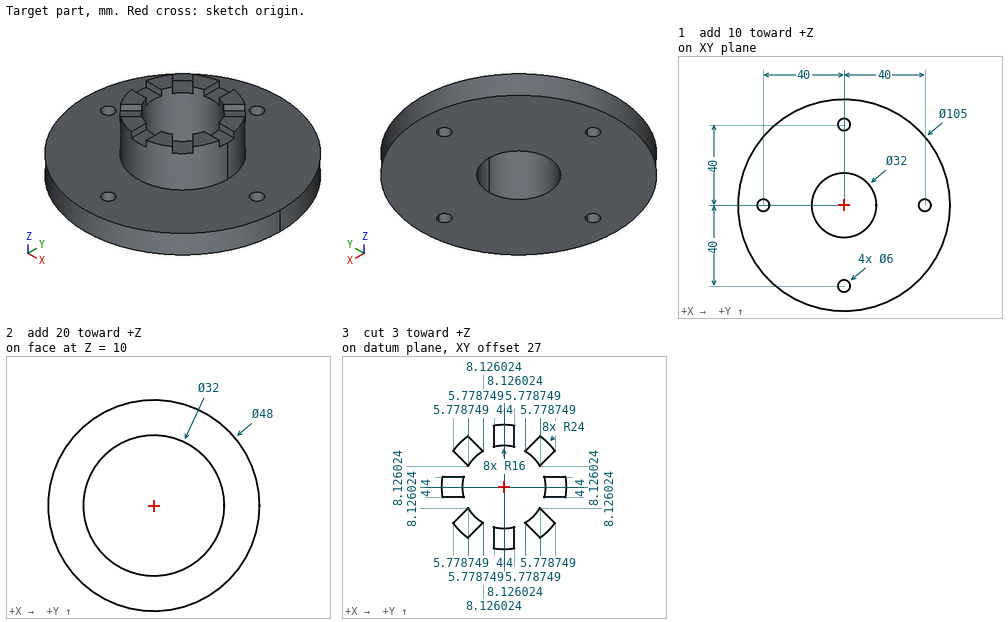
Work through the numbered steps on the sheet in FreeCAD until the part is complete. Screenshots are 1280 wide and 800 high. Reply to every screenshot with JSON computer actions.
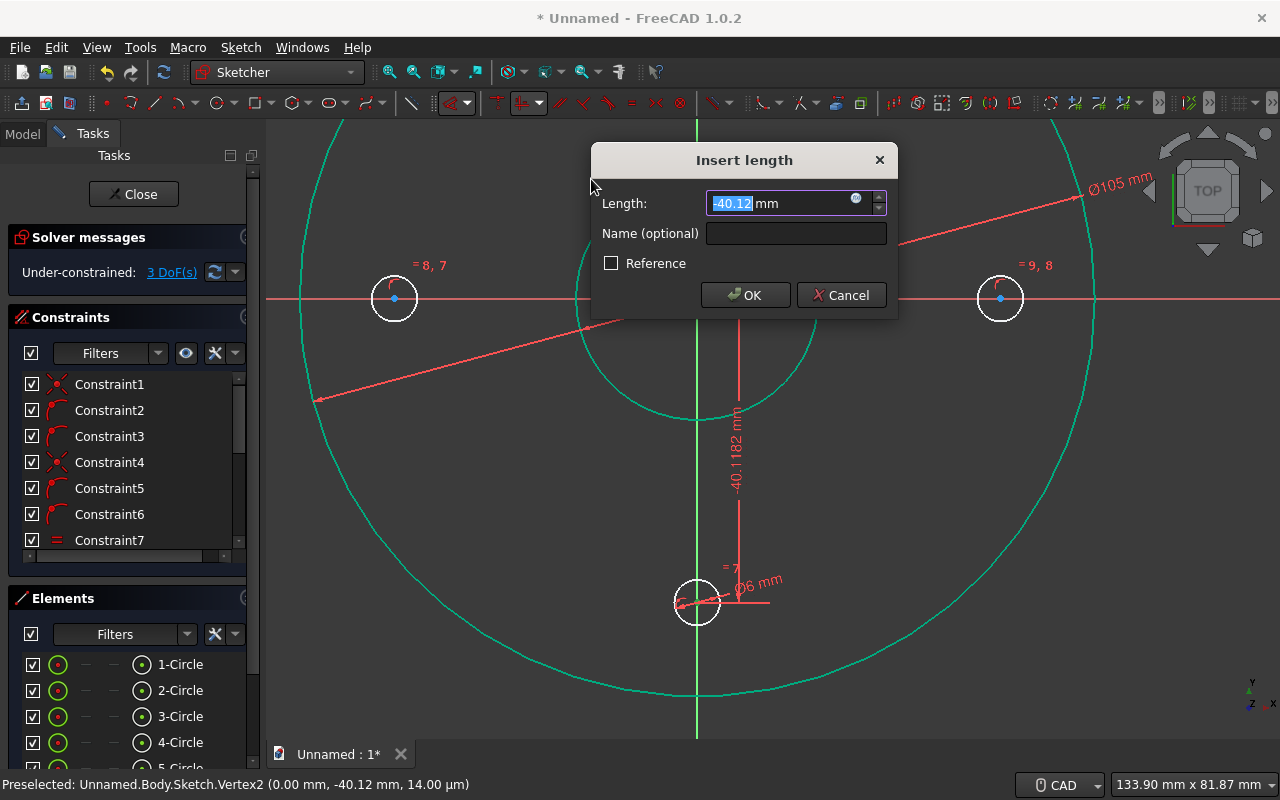
{"action": "type", "text": "-40"}
{"action": "key", "text": "Return"}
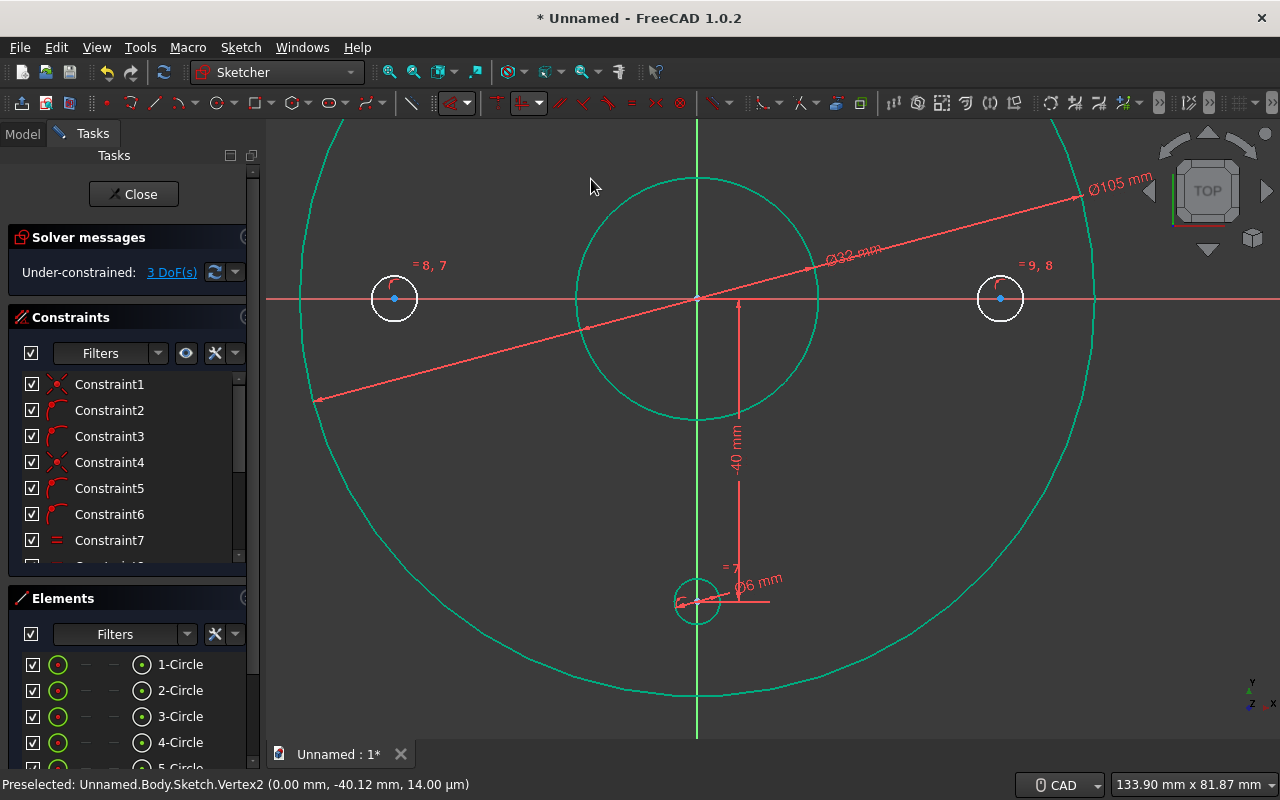
{"action": "left_click", "coordinate": [394, 299]}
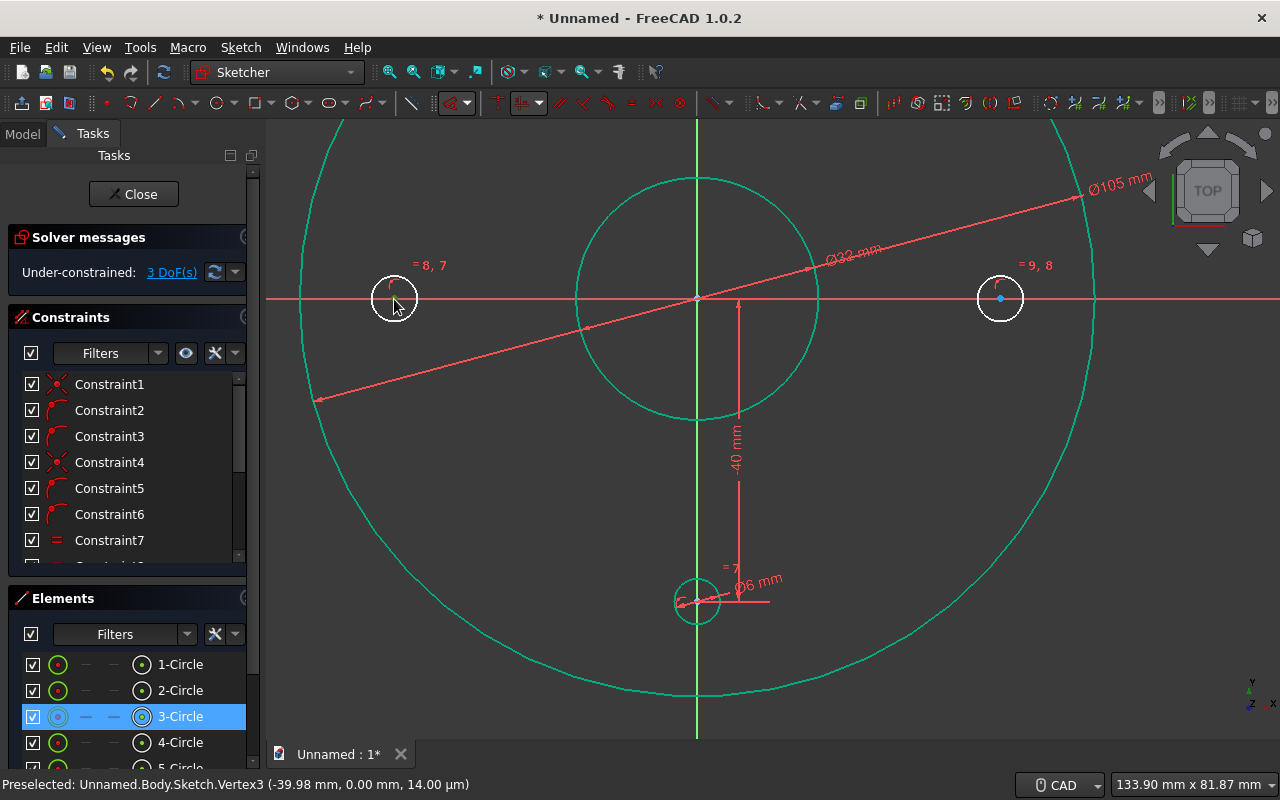
{"action": "left_click", "coordinate": [470, 104]}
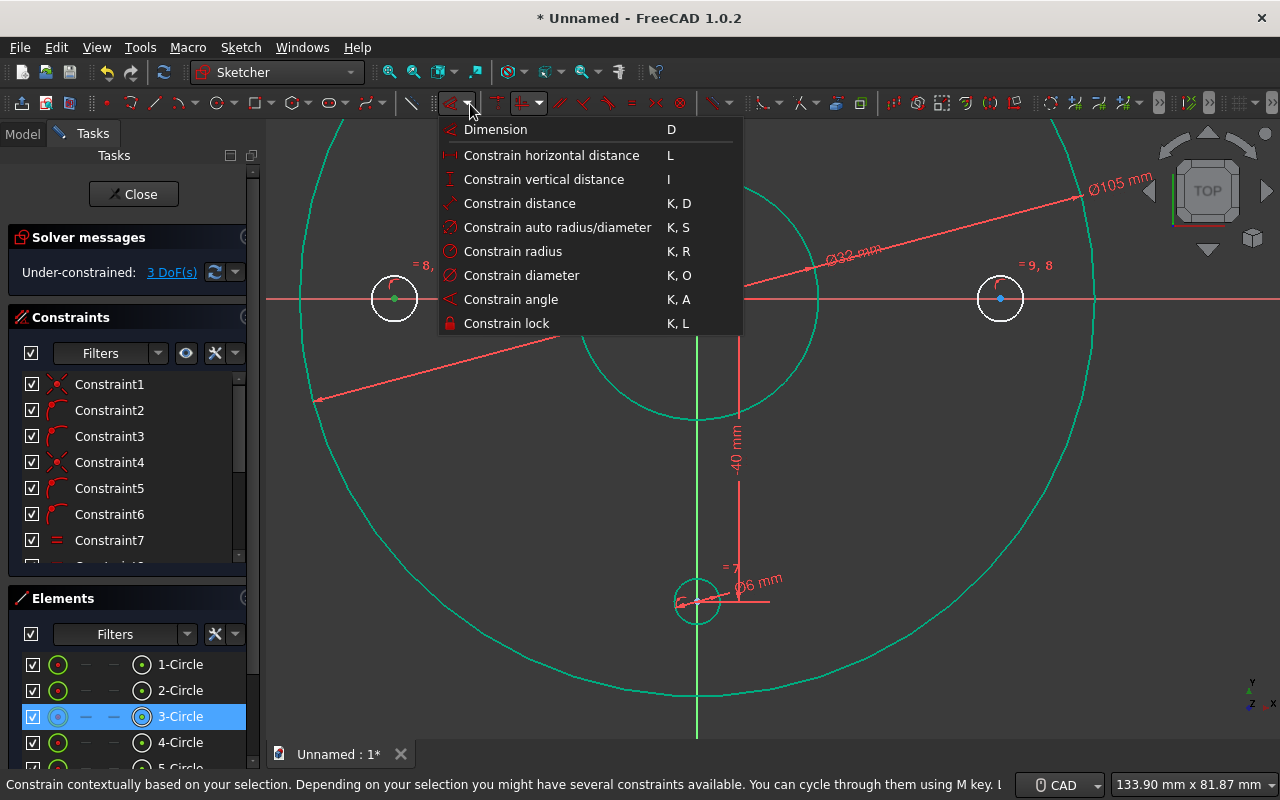
{"action": "left_click", "coordinate": [591, 155]}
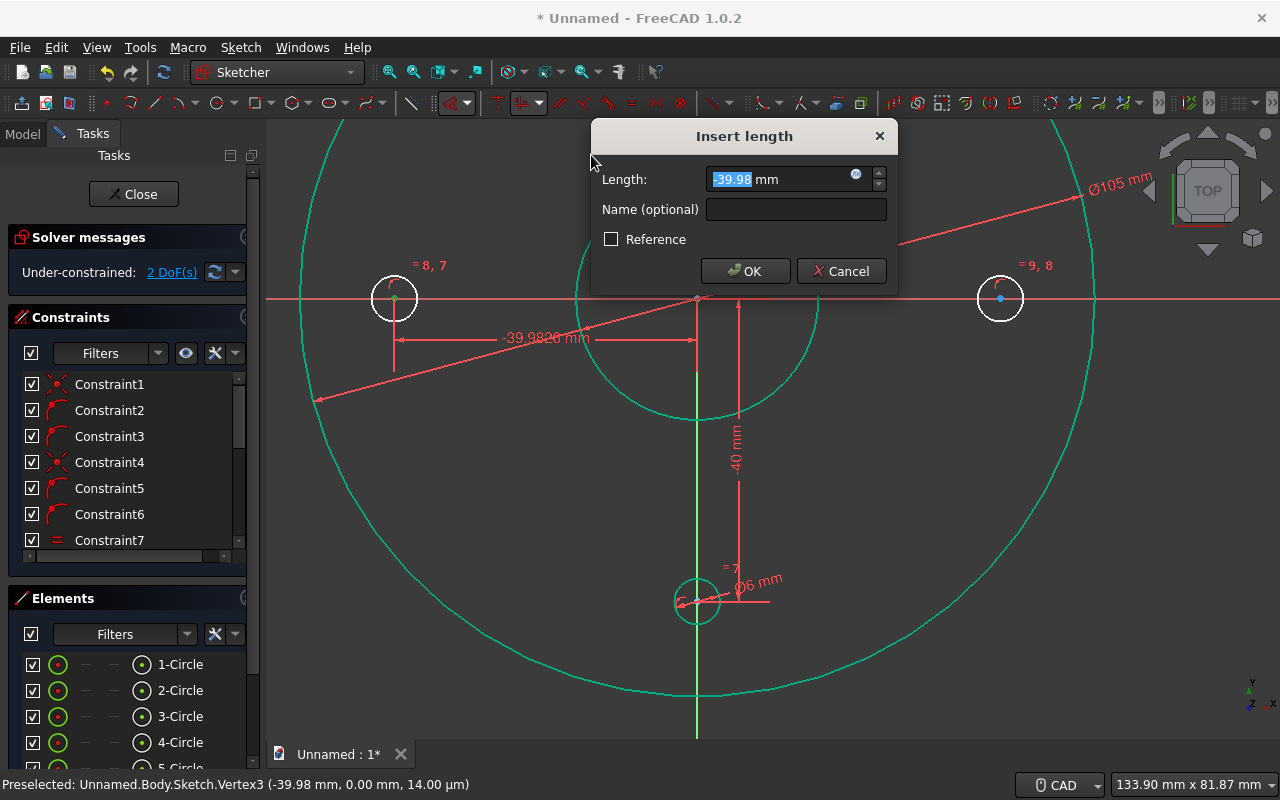
{"action": "type", "text": "-40"}
{"action": "key", "text": "Return"}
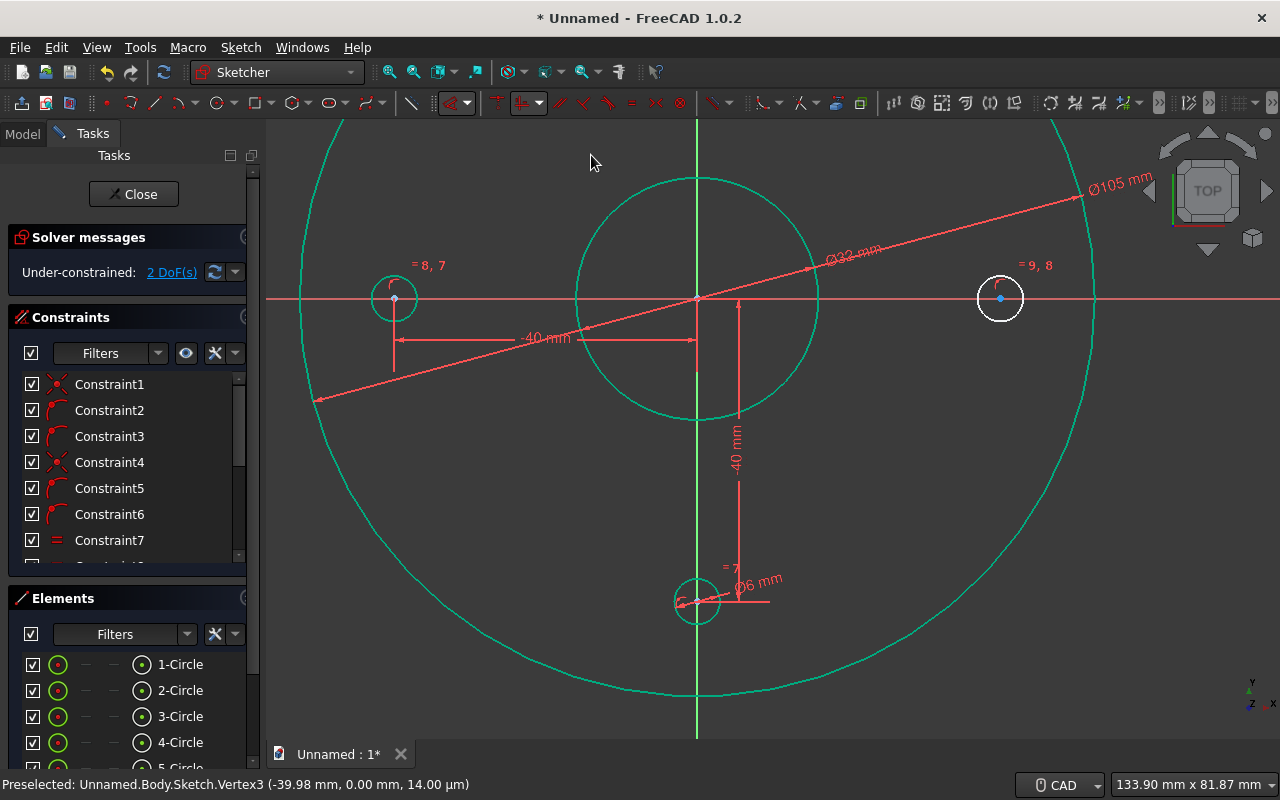
{"action": "left_click", "coordinate": [1000, 299]}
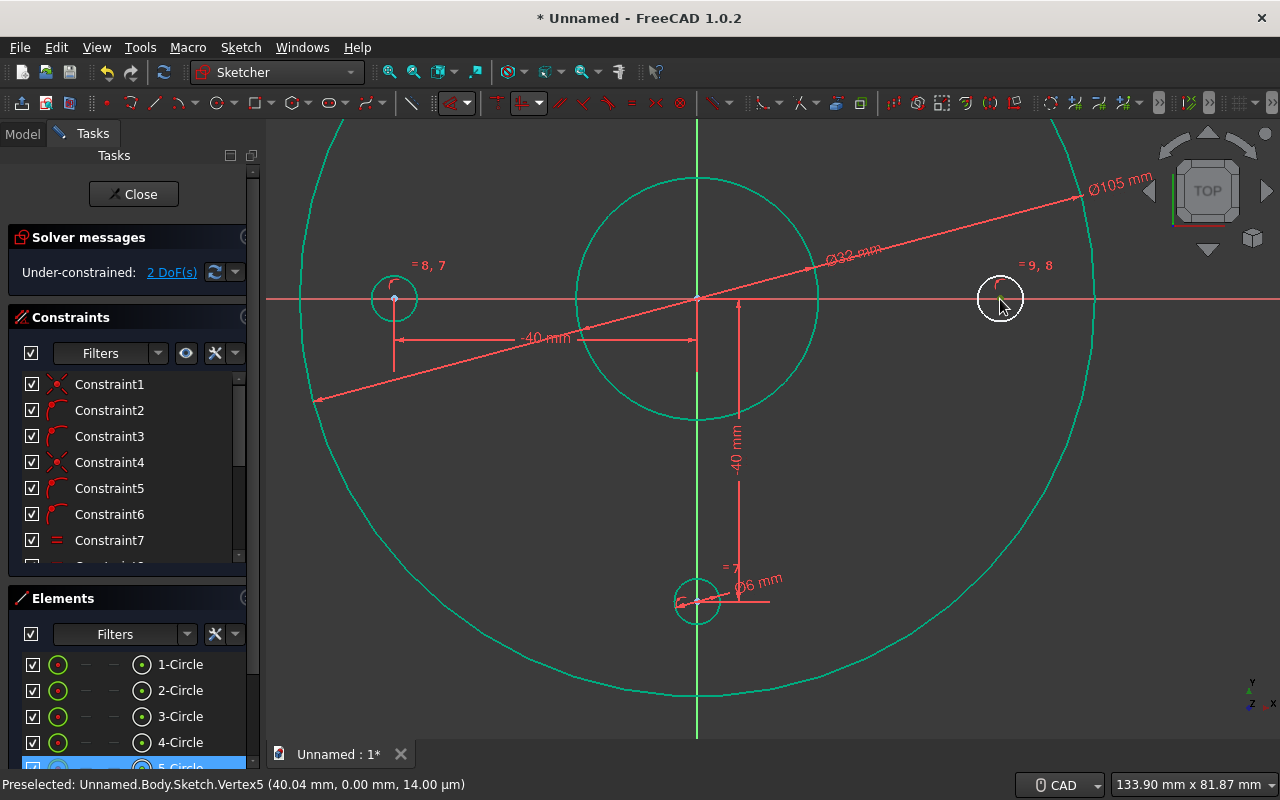
{"action": "left_click", "coordinate": [470, 104]}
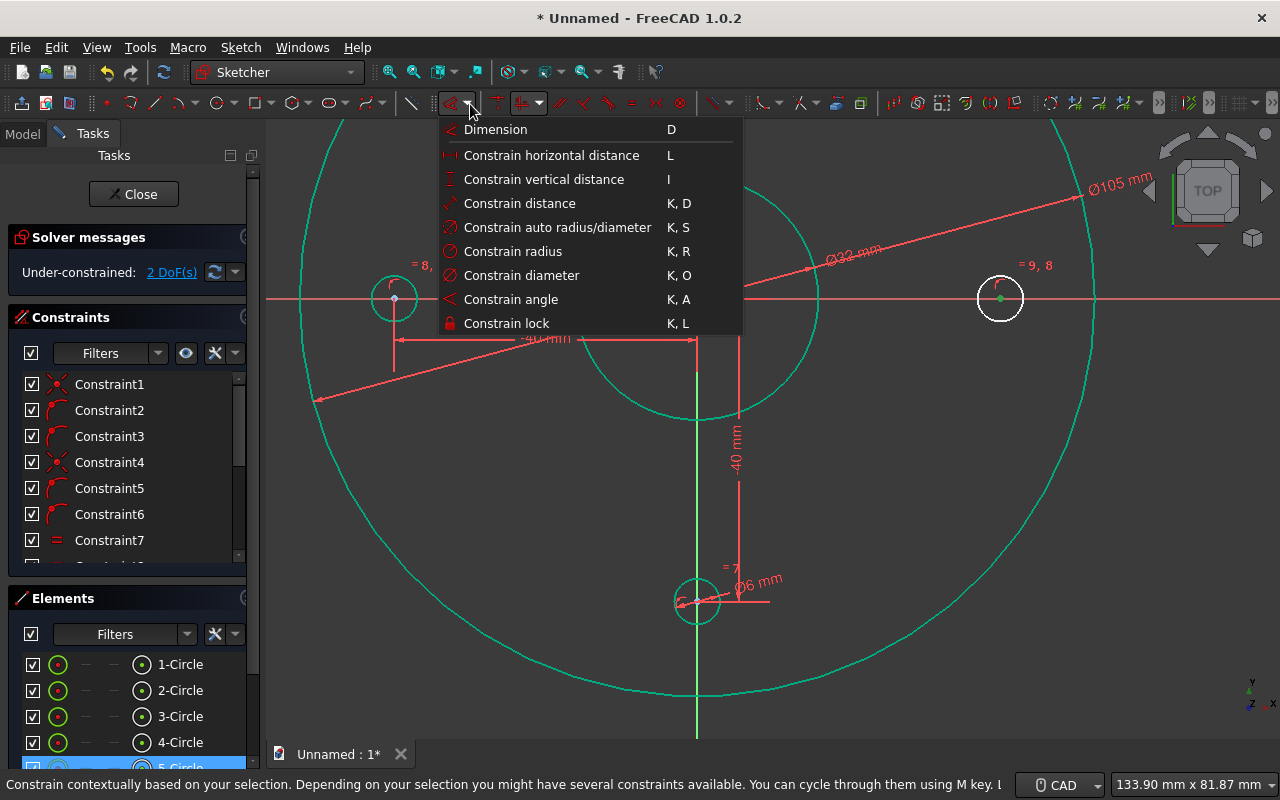
{"action": "left_click", "coordinate": [591, 155]}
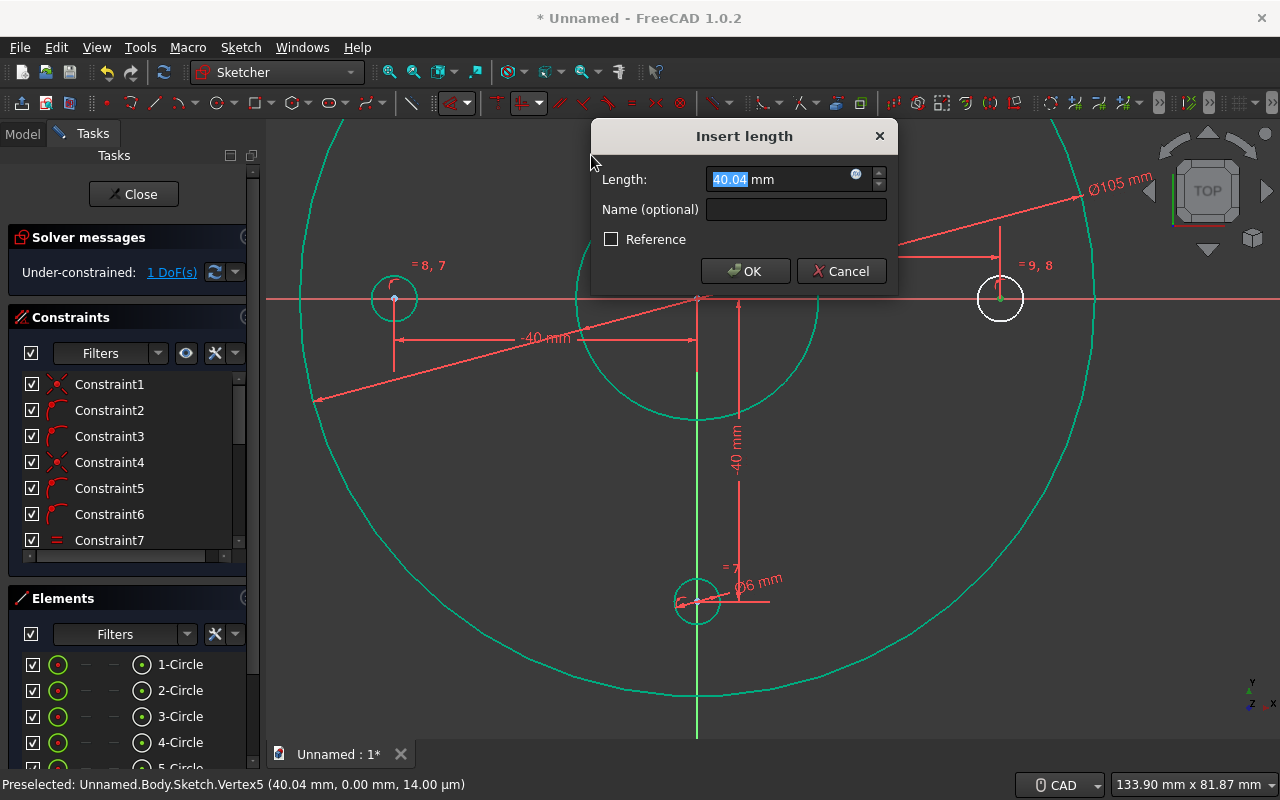
{"action": "type", "text": "40"}
{"action": "key", "text": "Return"}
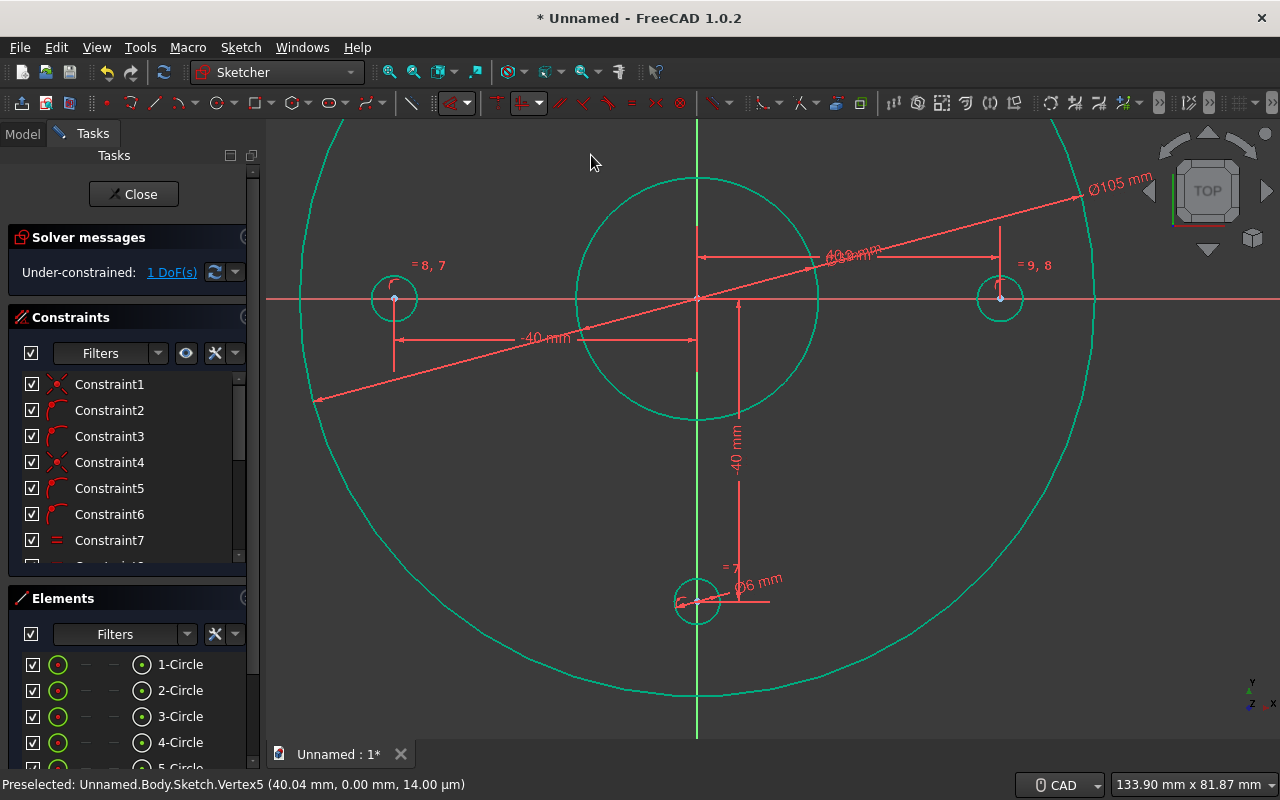
{"action": "scroll", "coordinate": [713, 587], "scroll_direction": "down", "scroll_amount": 3}